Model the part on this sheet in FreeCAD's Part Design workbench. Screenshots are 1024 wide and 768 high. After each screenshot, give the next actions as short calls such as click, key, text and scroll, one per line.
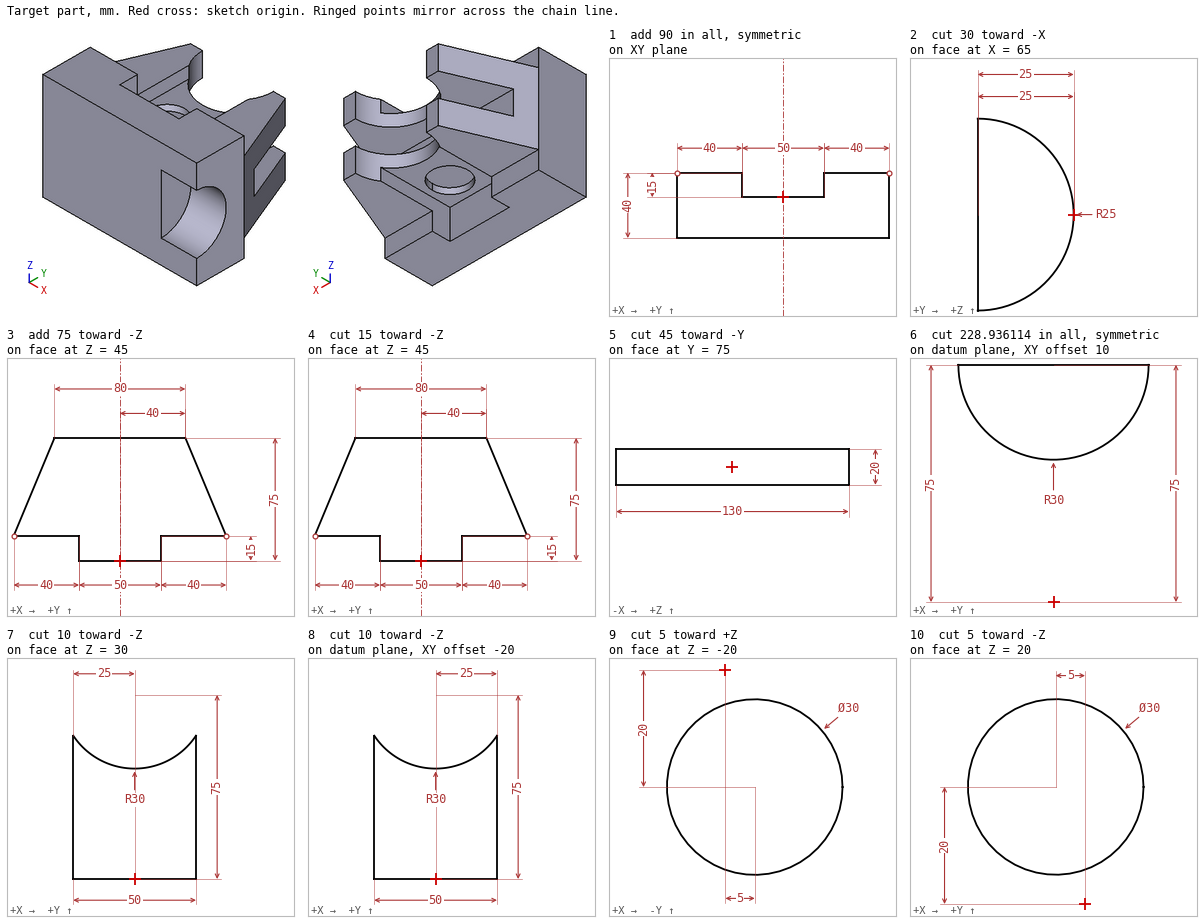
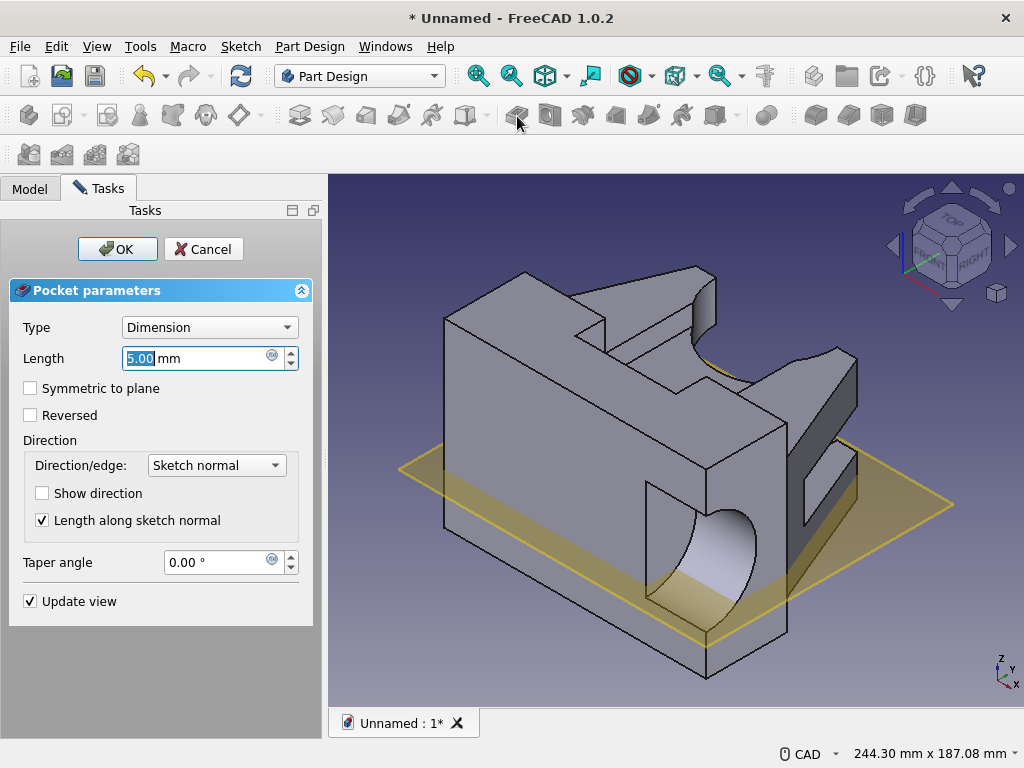
text(10)
key(Tab)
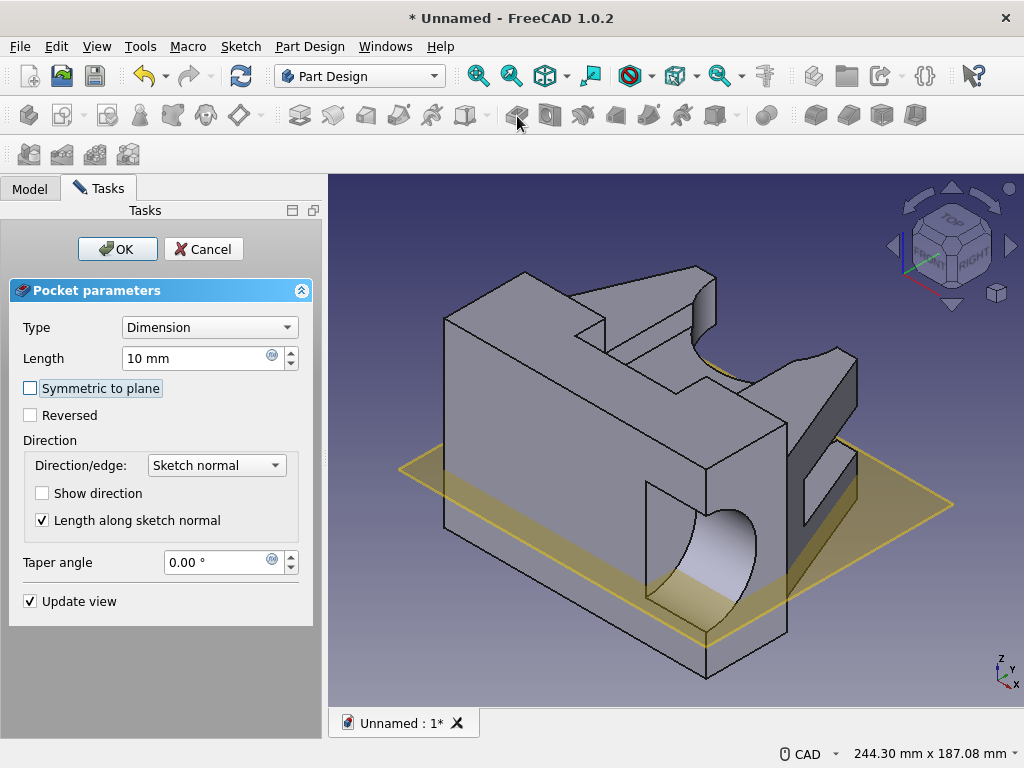
click(118, 249)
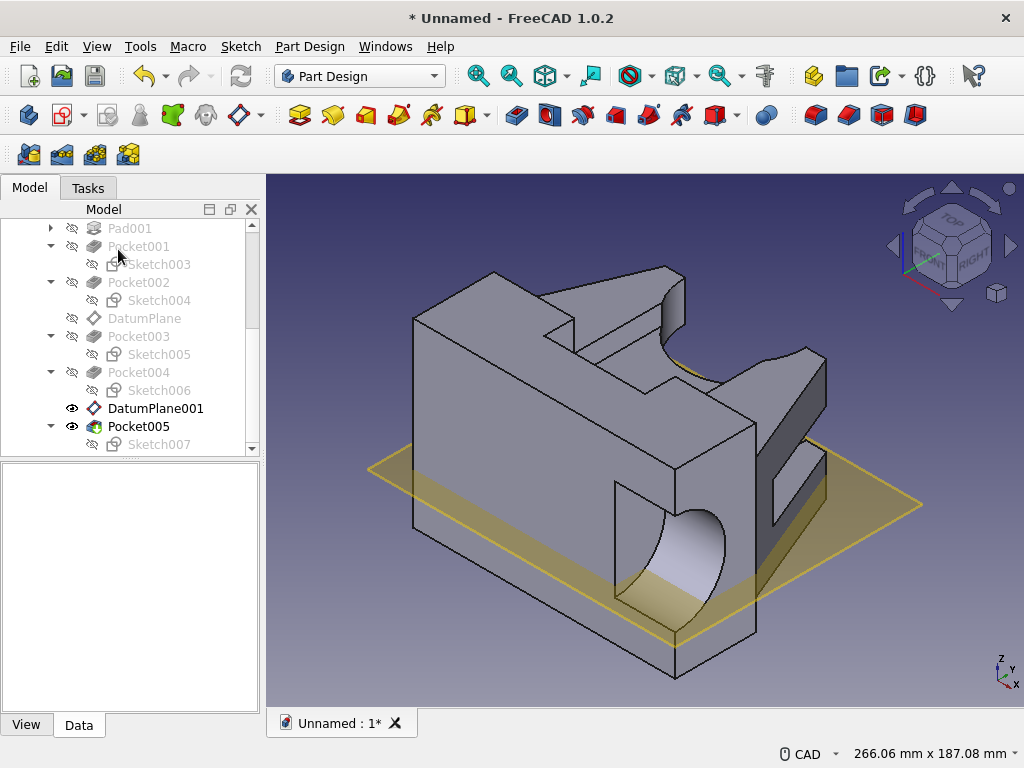
click(117, 408)
key(space)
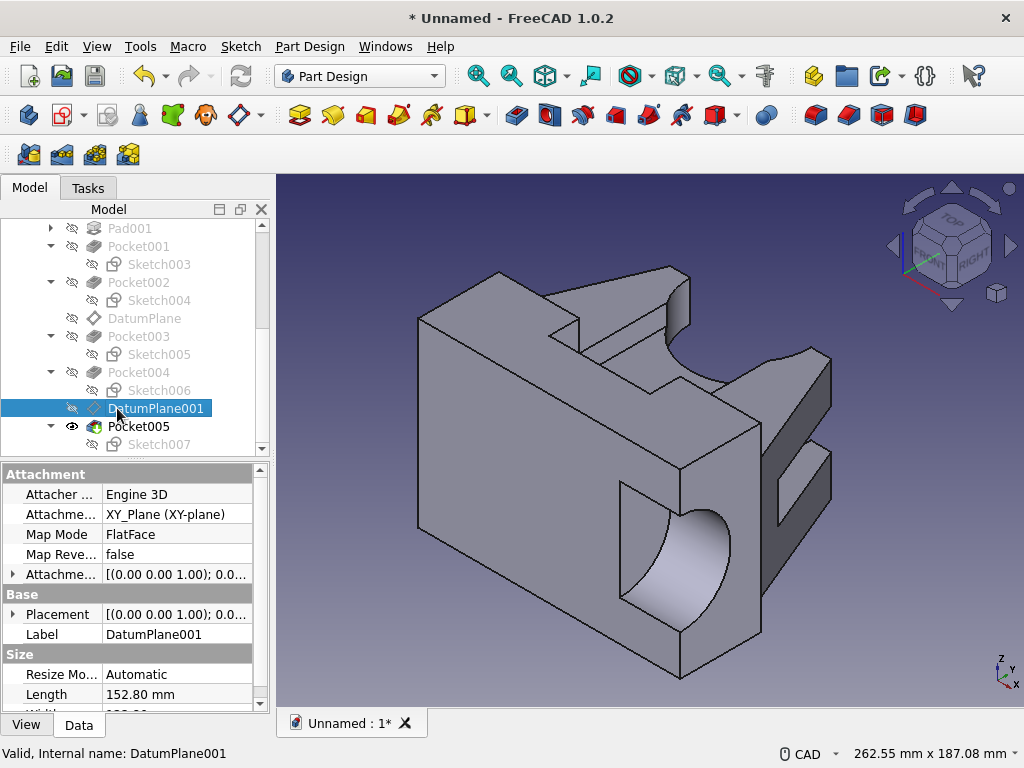
key(5)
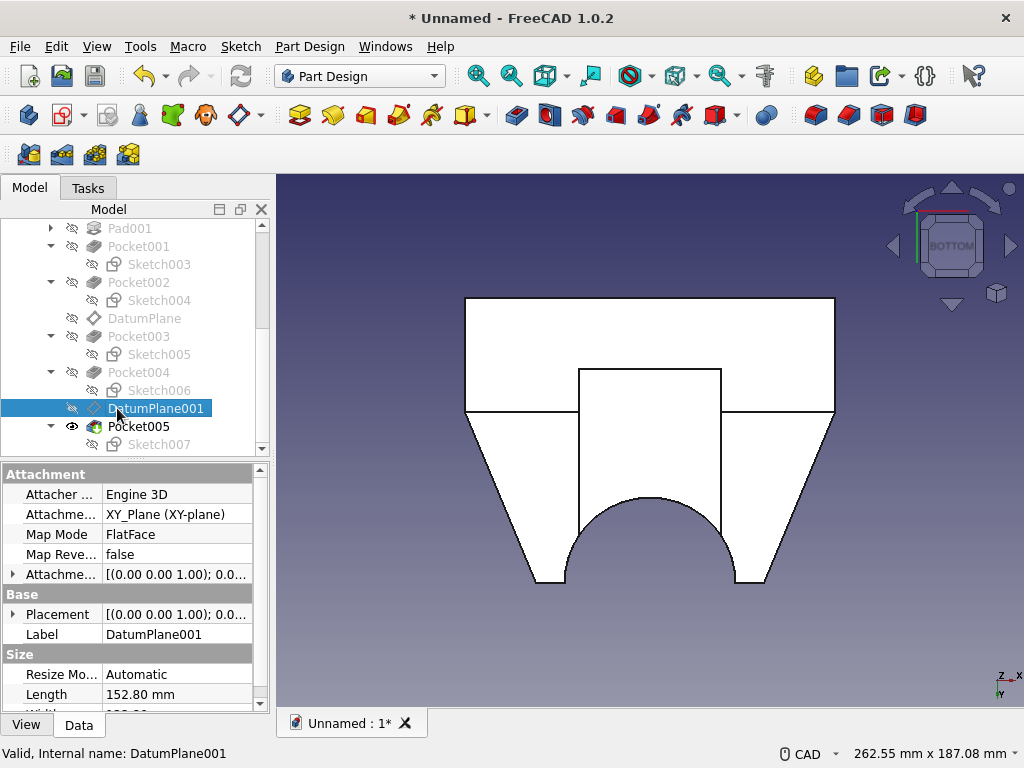
click(650, 428)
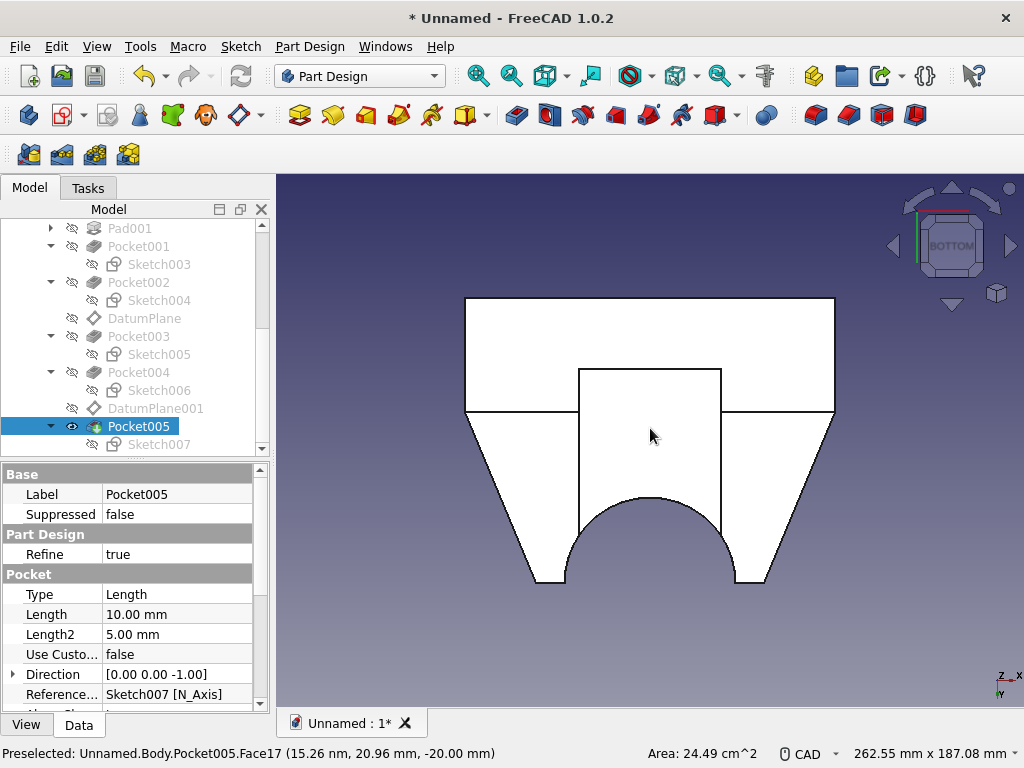
click(62, 116)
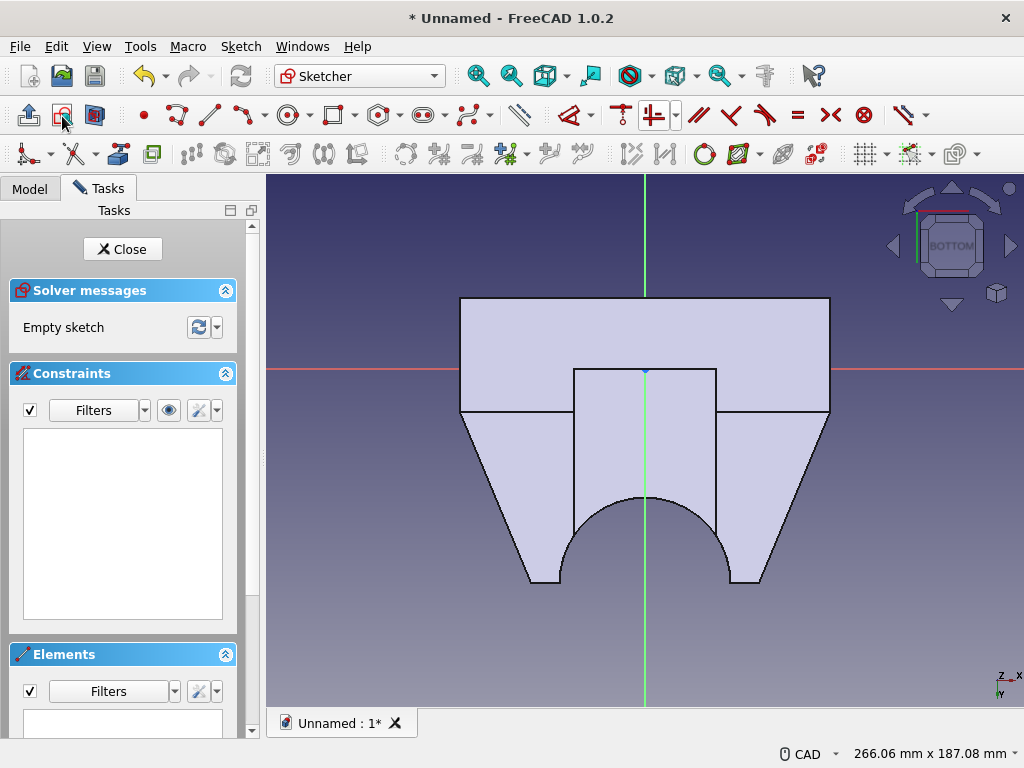
scroll(695, 410, up, 6)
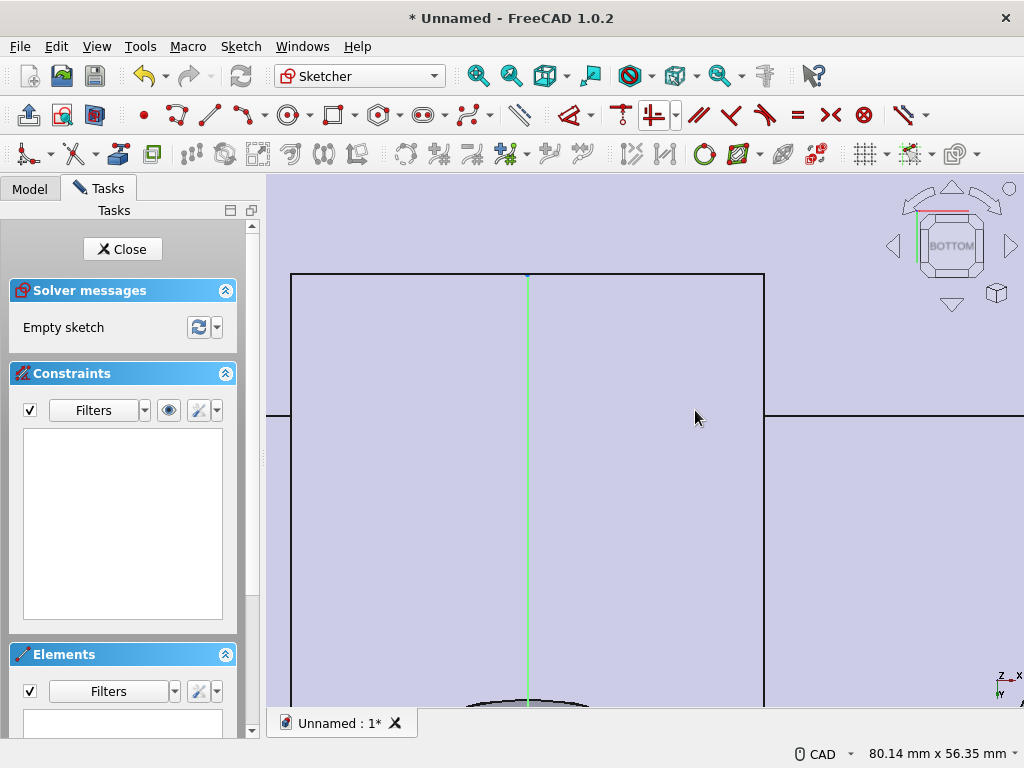
key(g)
key(c)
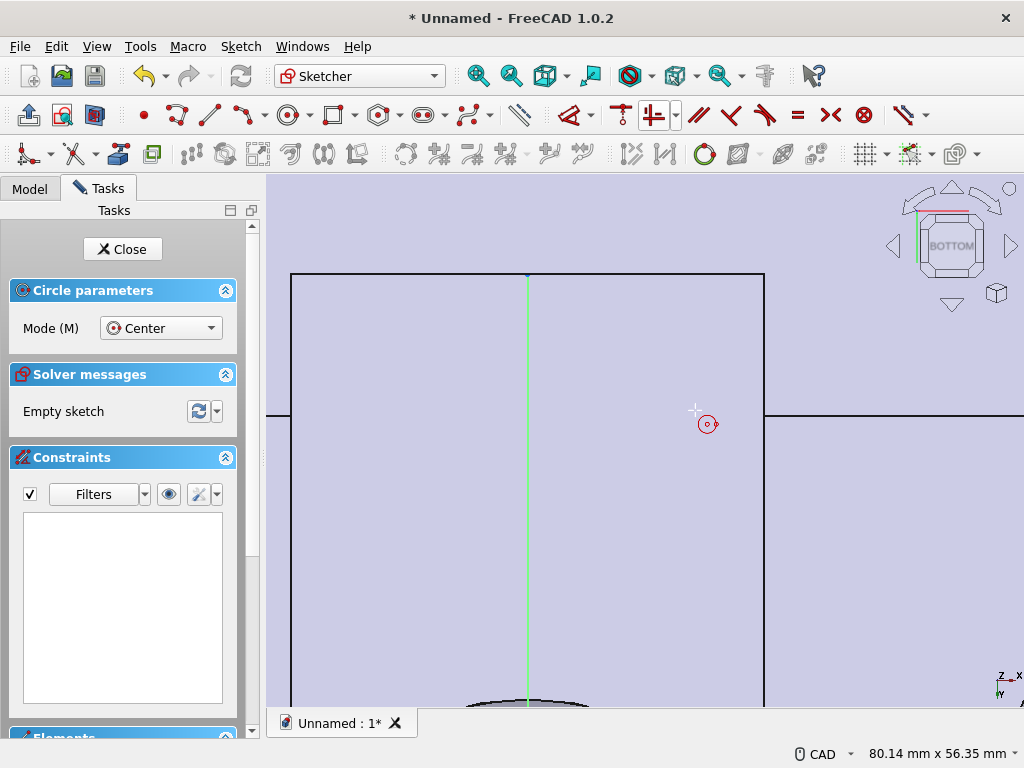
click(575, 463)
click(675, 363)
key(Escape)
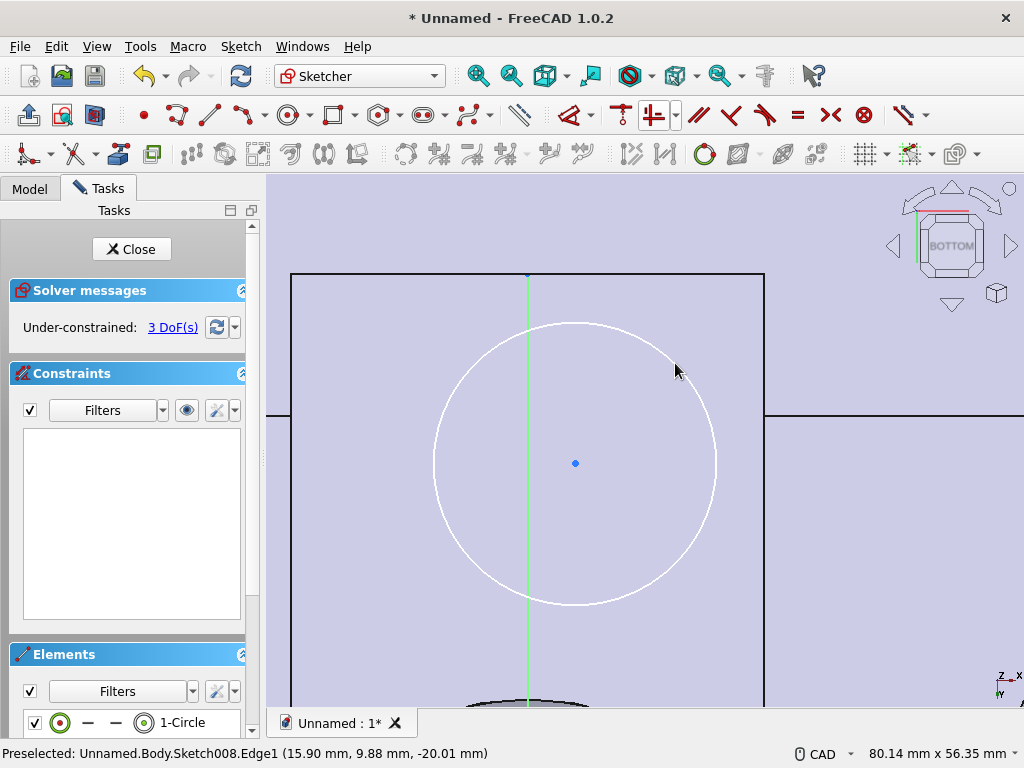
key(d)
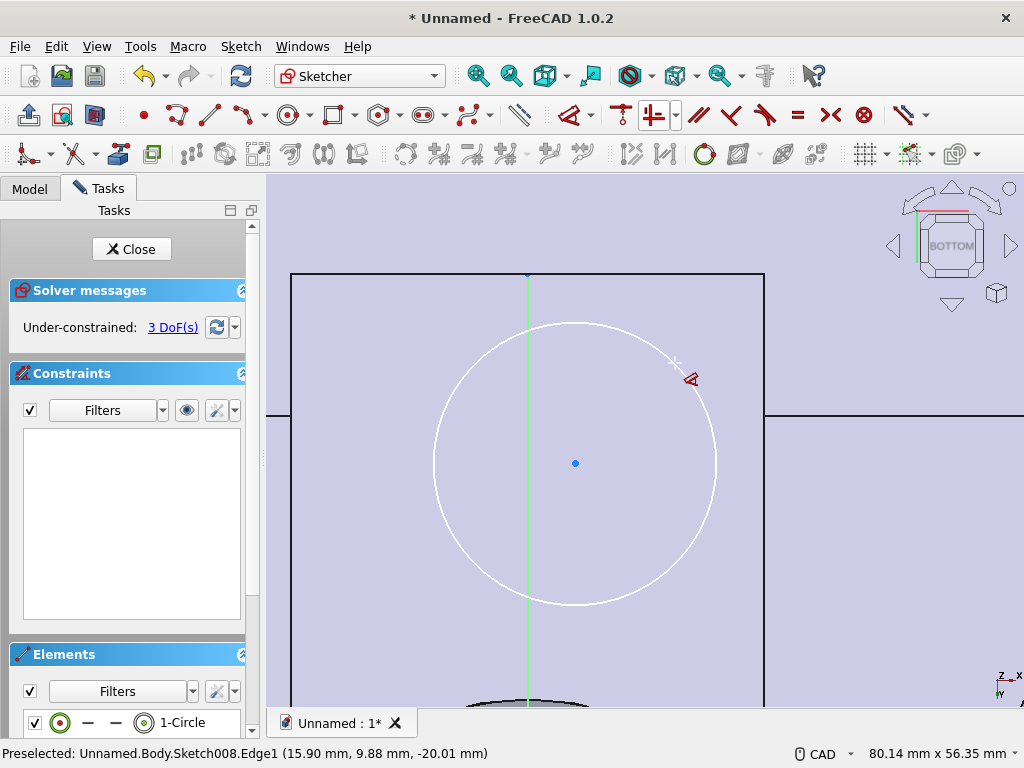
click(675, 364)
click(698, 341)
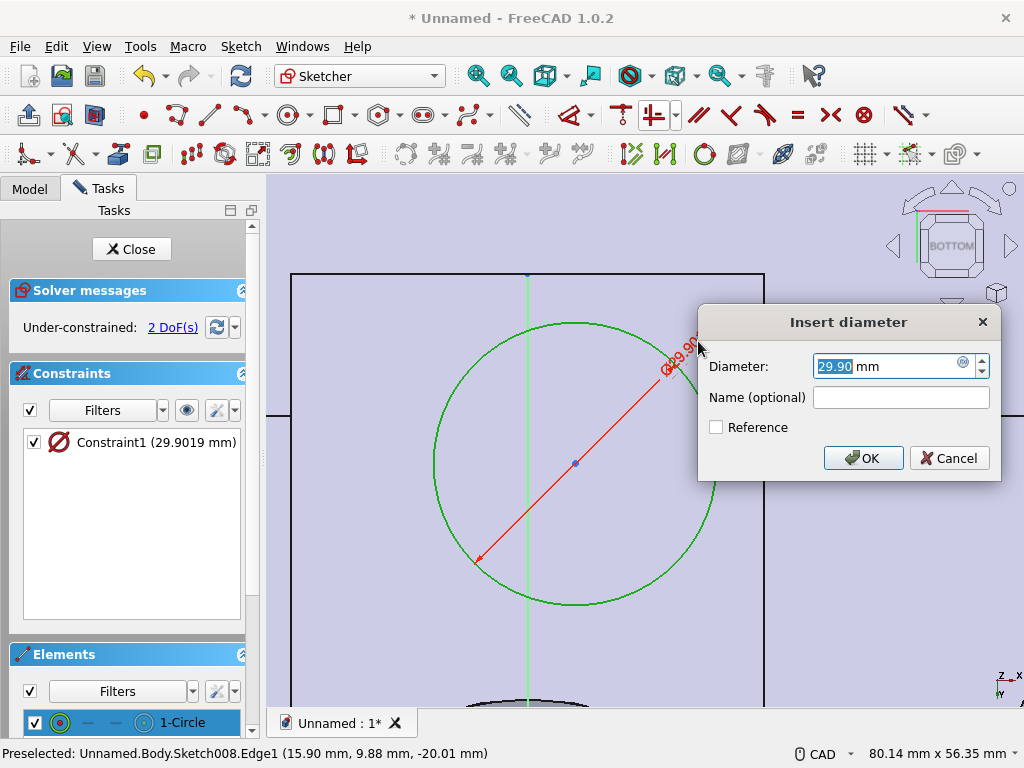
text(30)
key(Return)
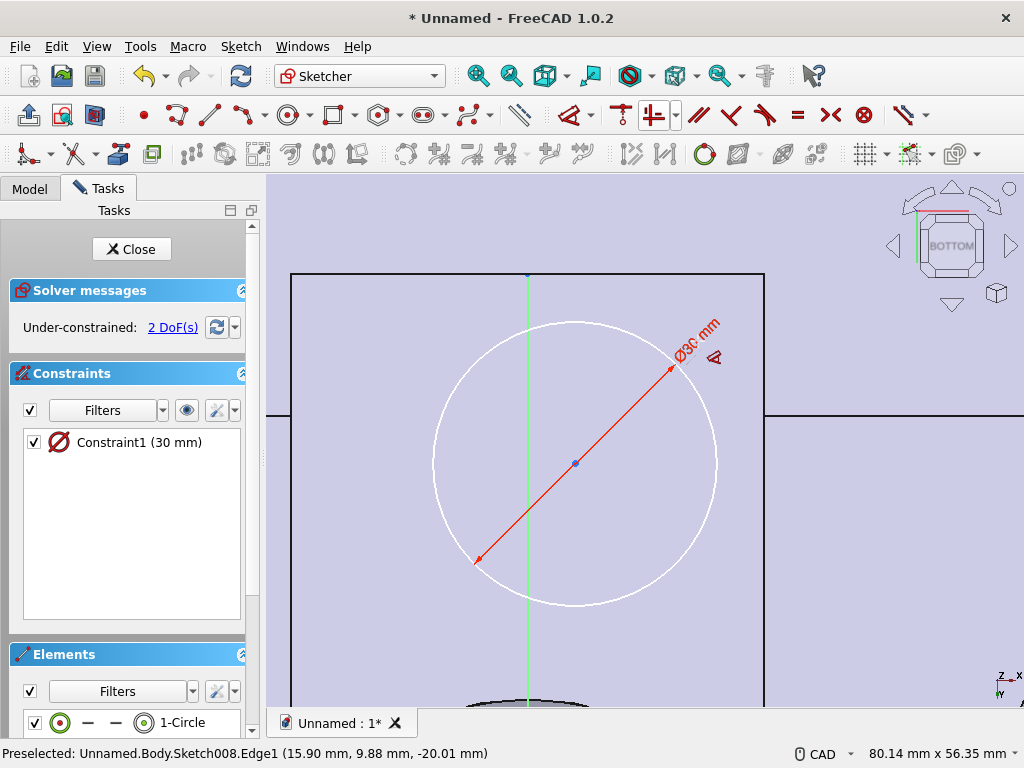
click(575, 464)
click(551, 240)